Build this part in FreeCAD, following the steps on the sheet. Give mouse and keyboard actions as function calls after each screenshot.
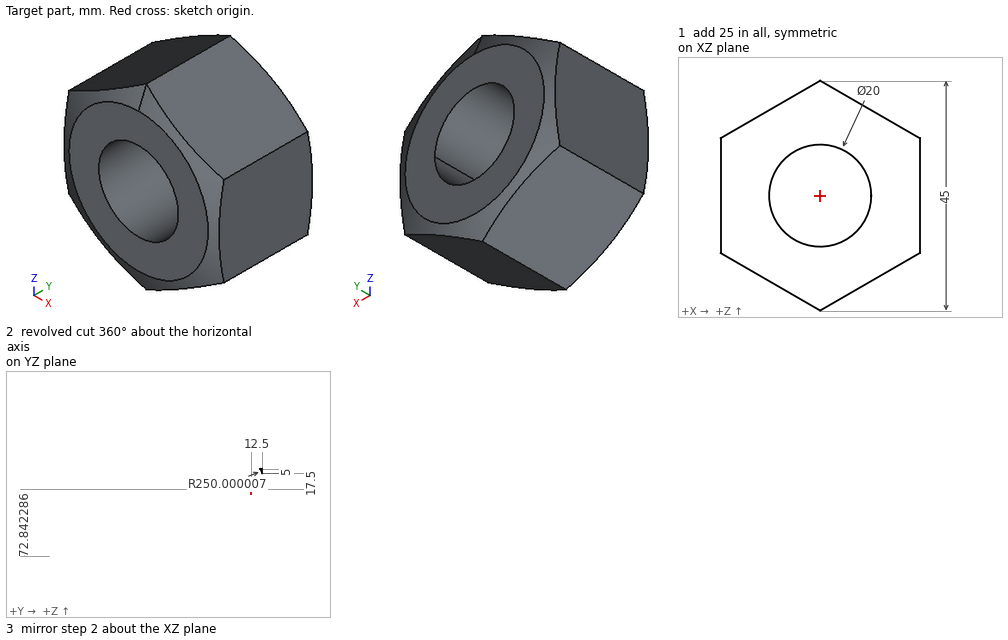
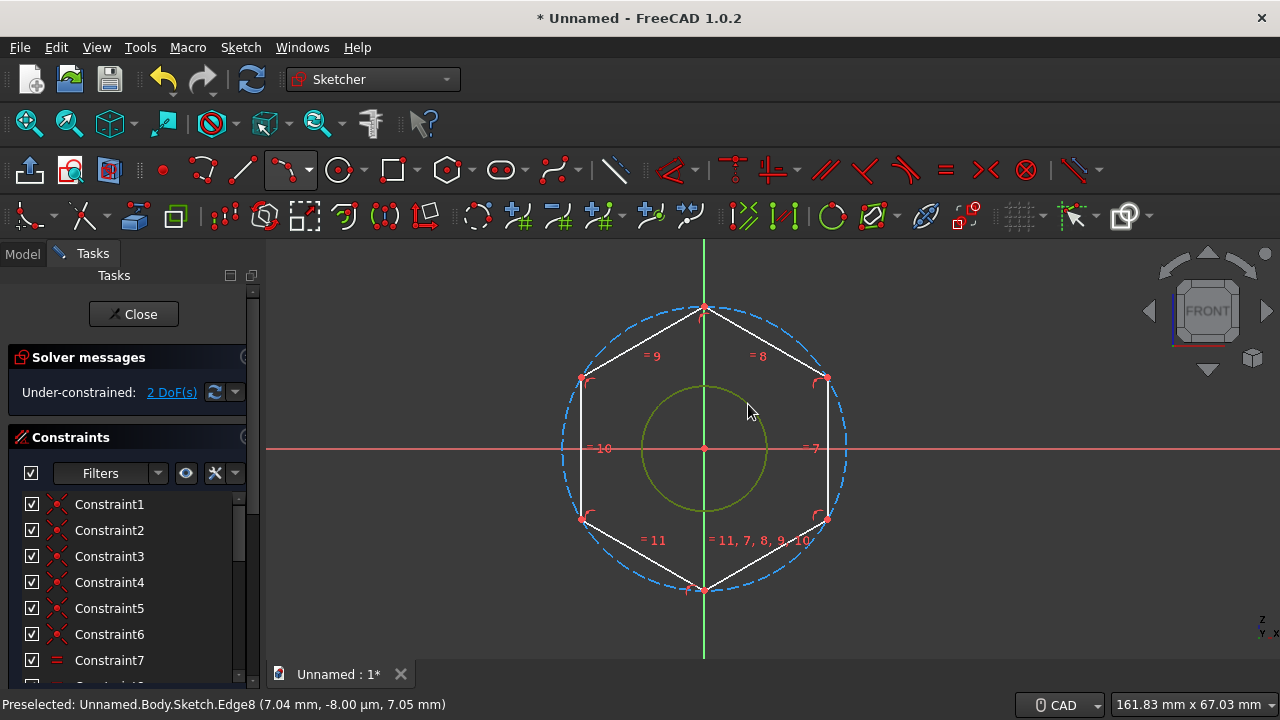
key(k)
key(o)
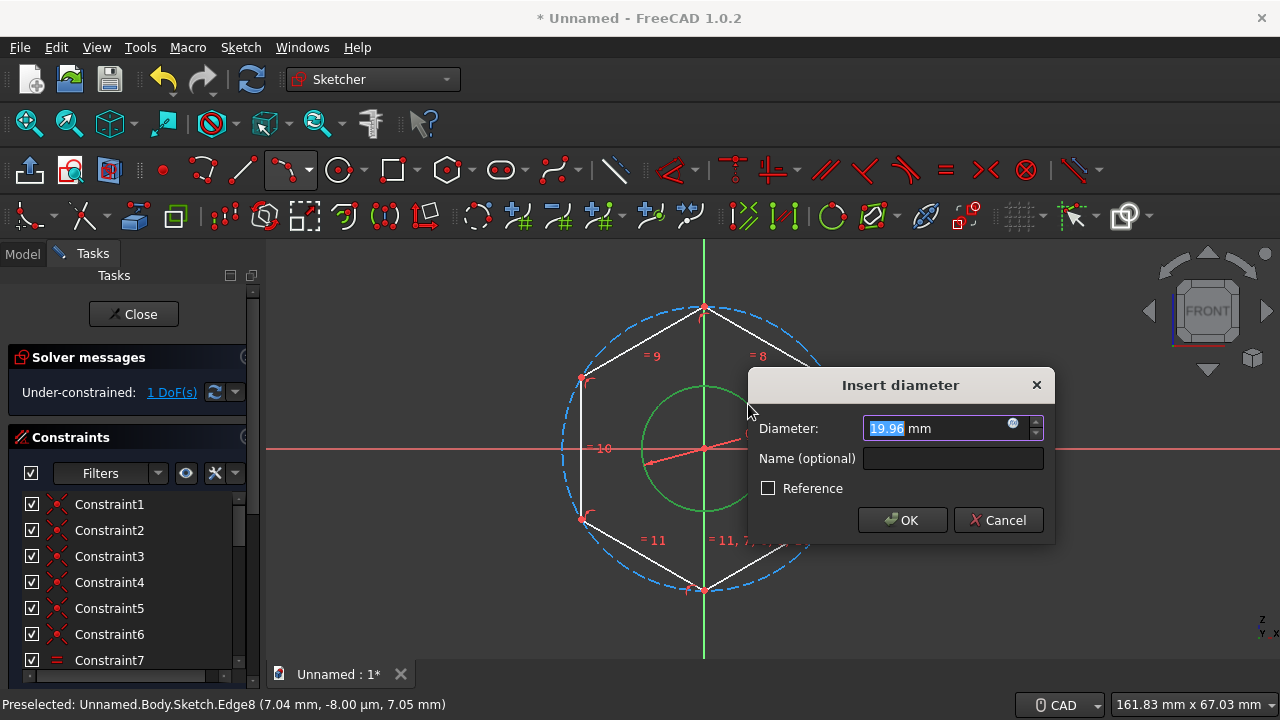
text(20)
key(Return)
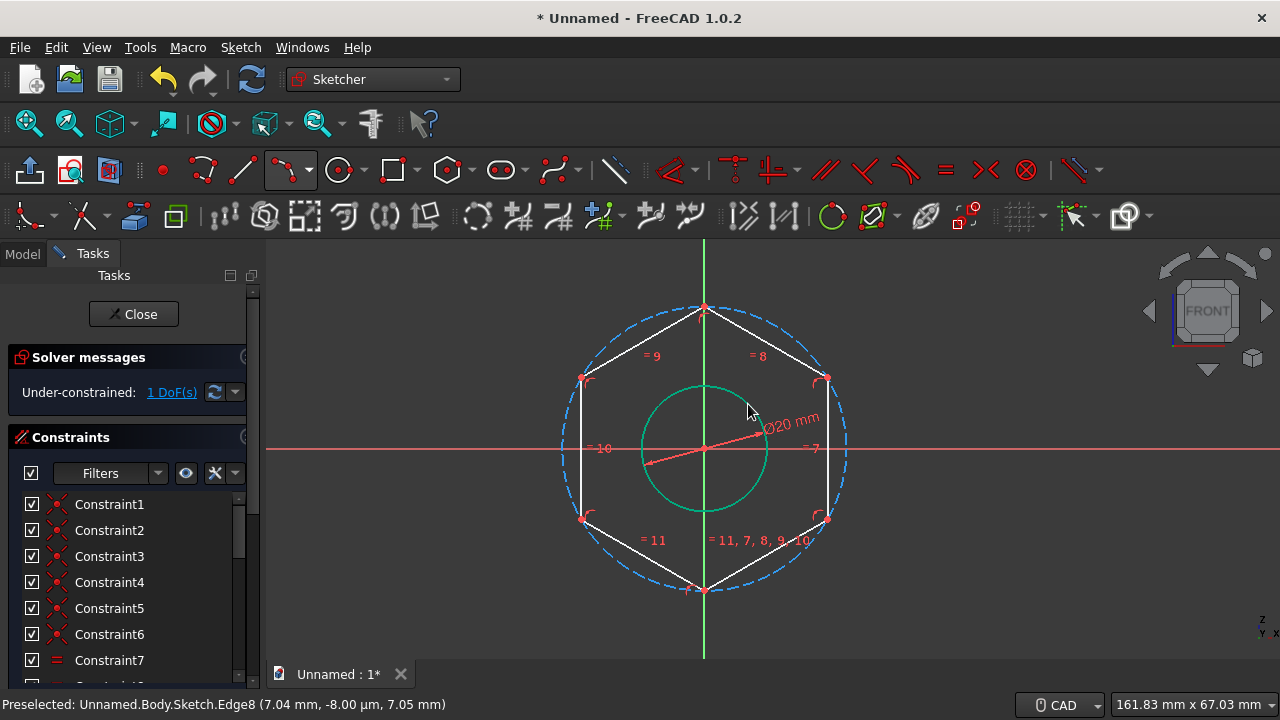
click(704, 591)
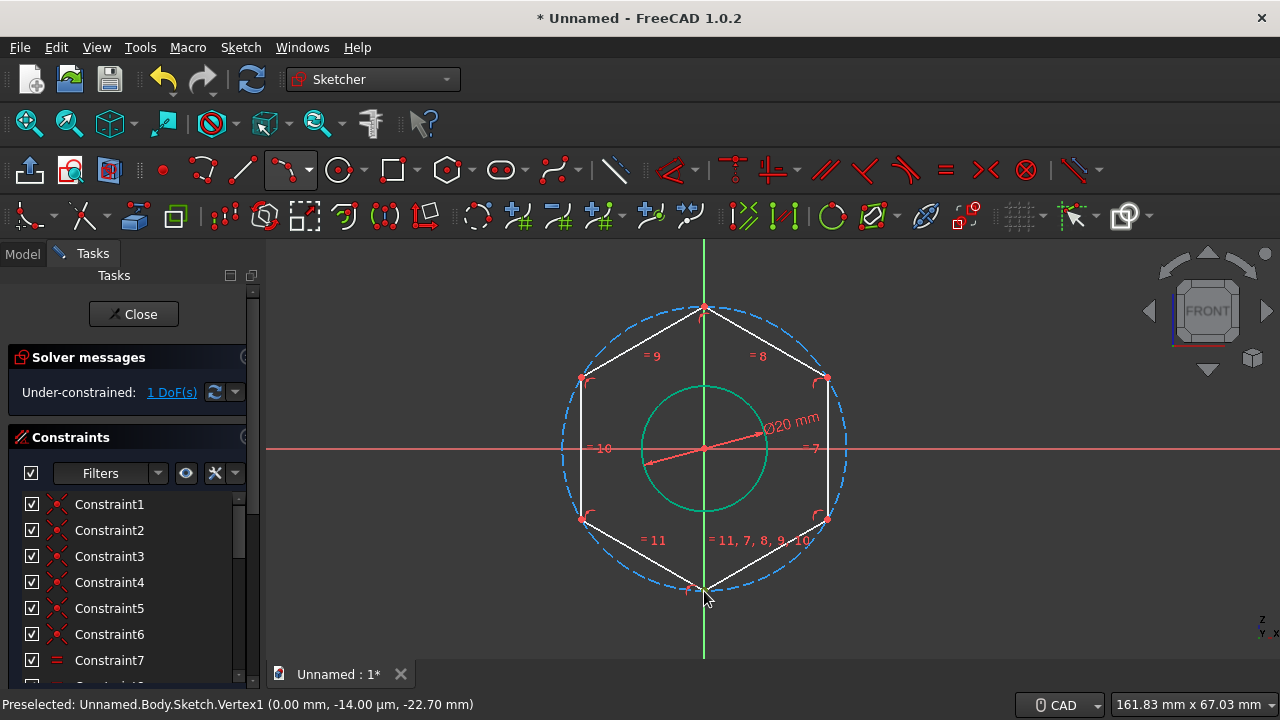
click(704, 307)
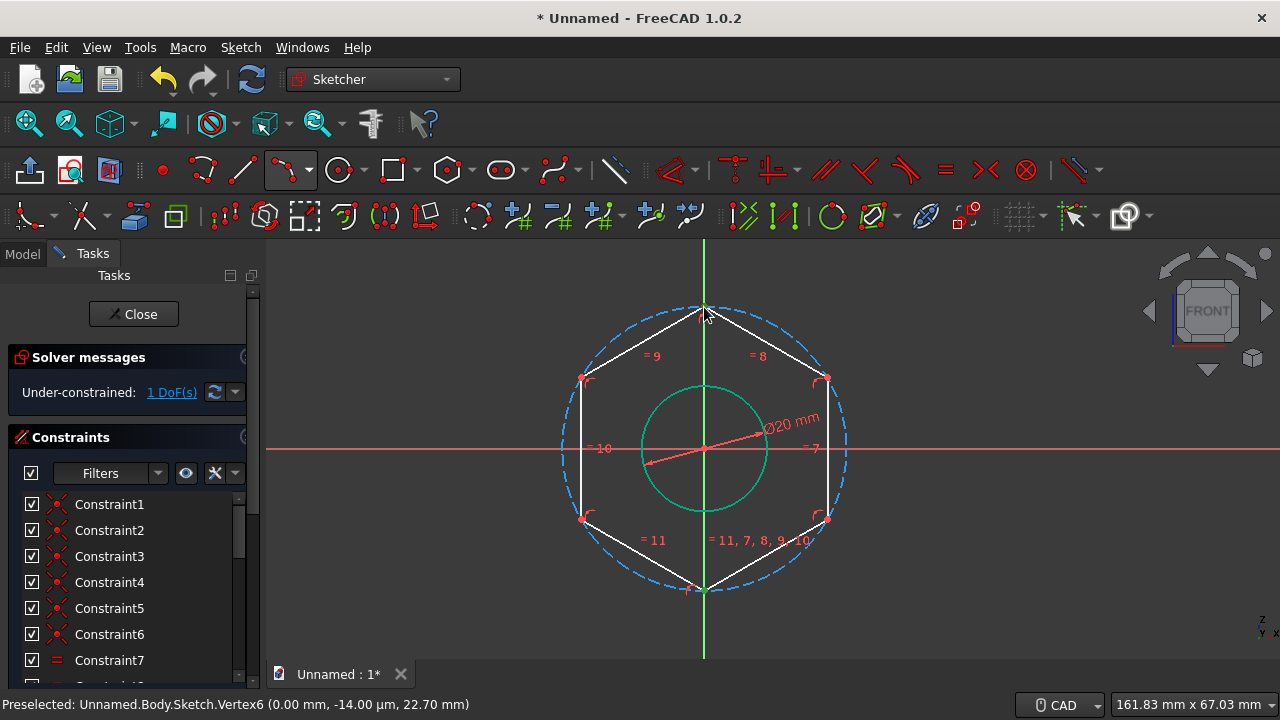
click(698, 170)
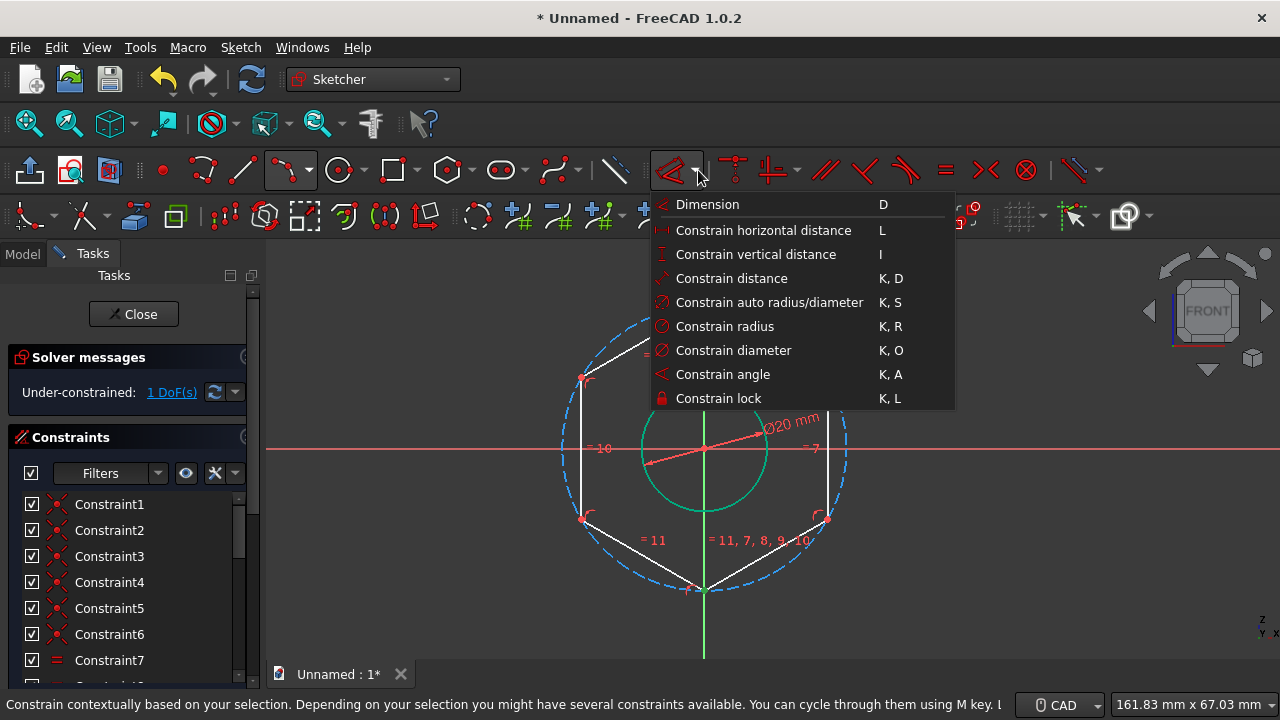
click(803, 254)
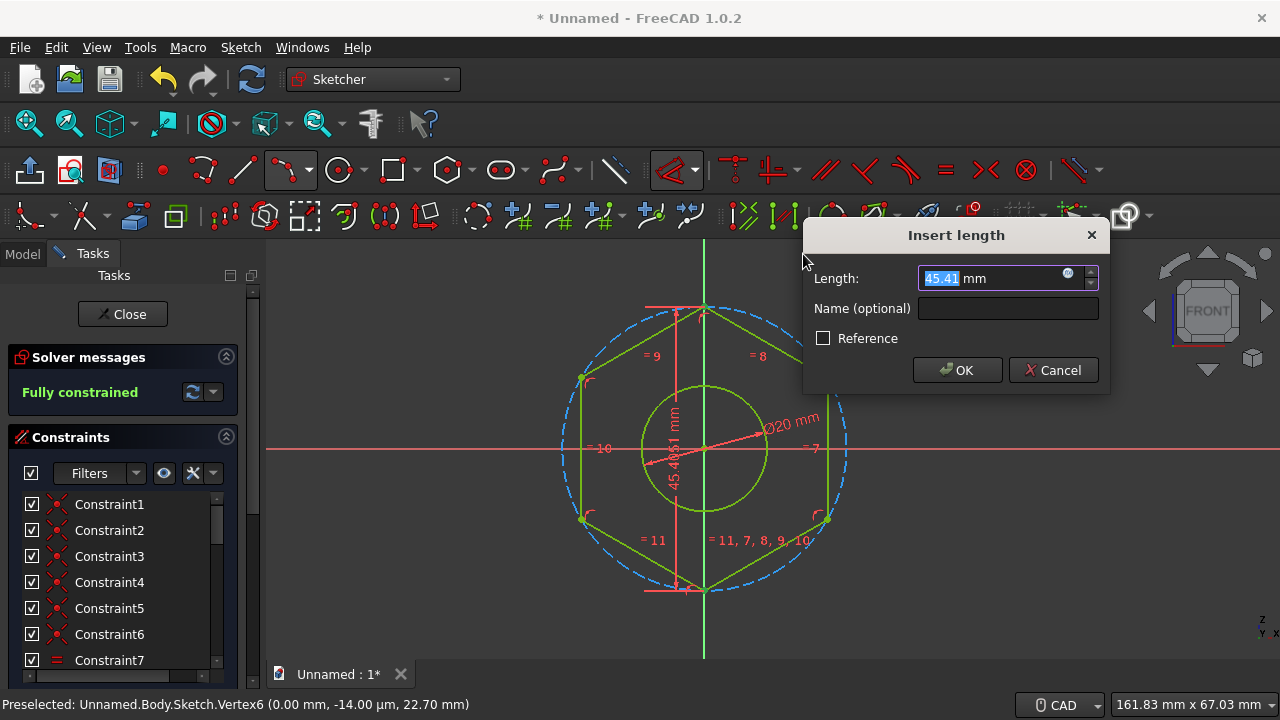
text(45)
key(Return)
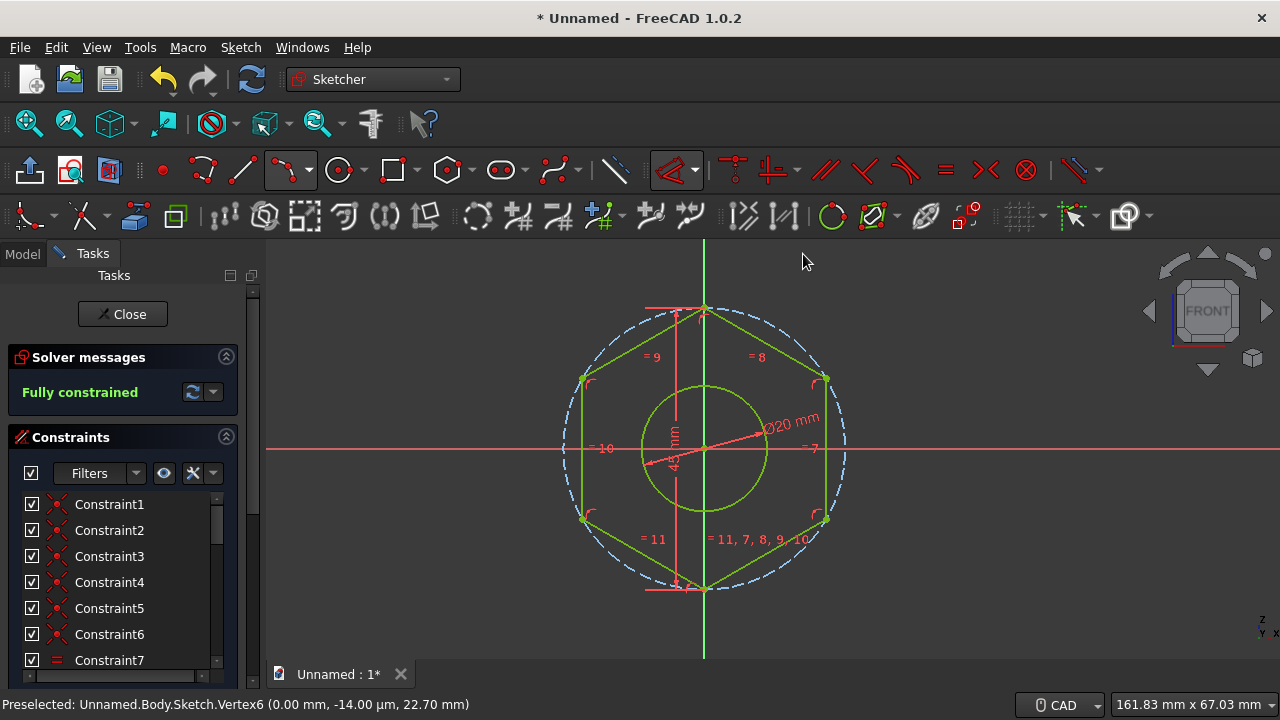
click(123, 314)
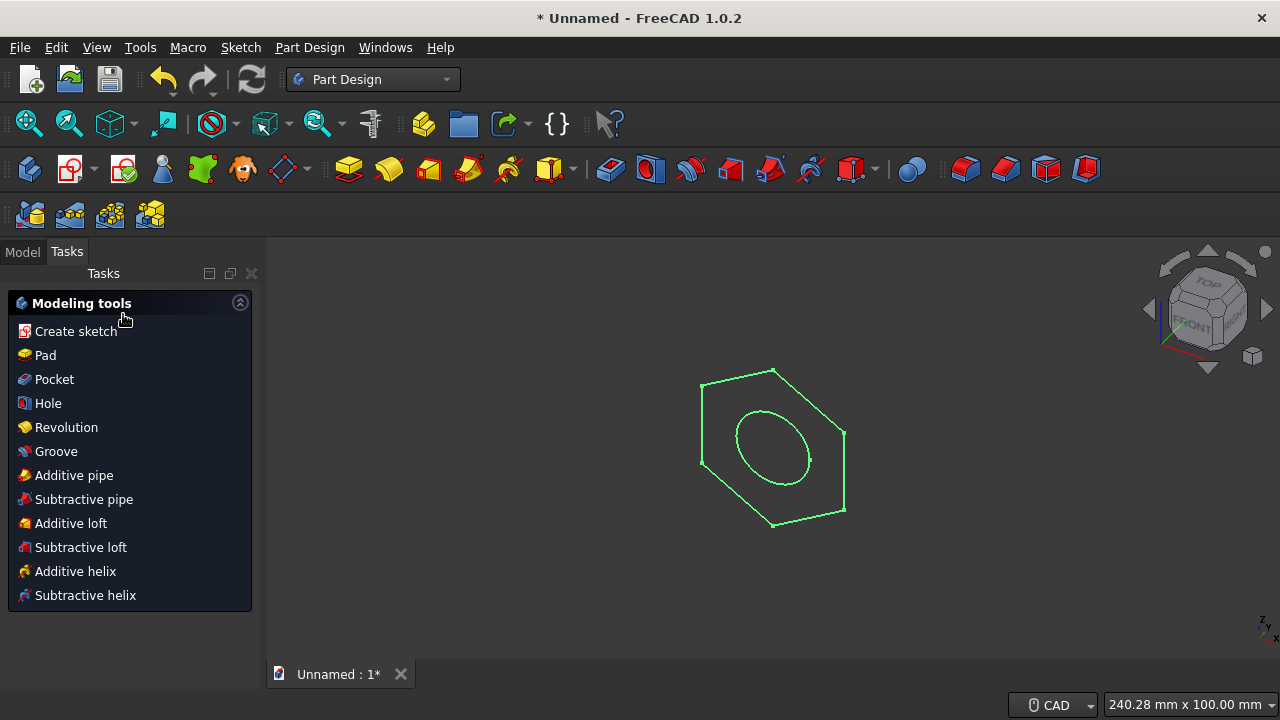
click(350, 170)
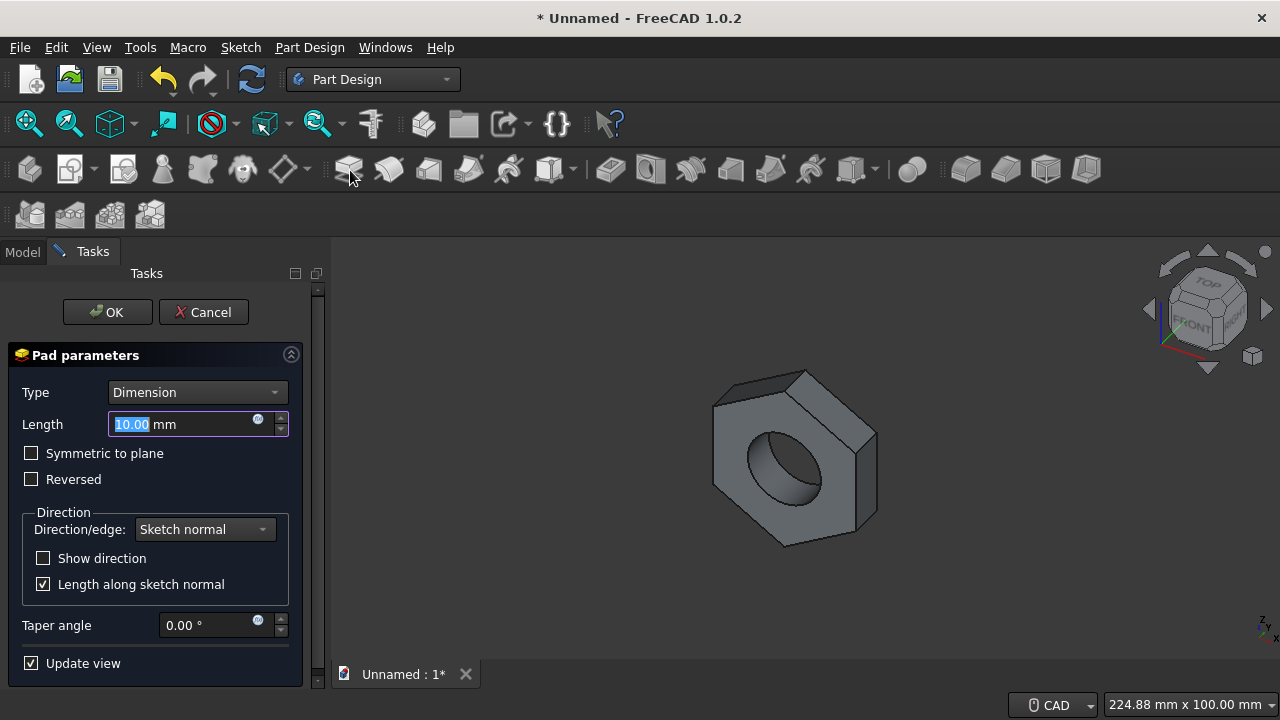
text(25)
key(Tab)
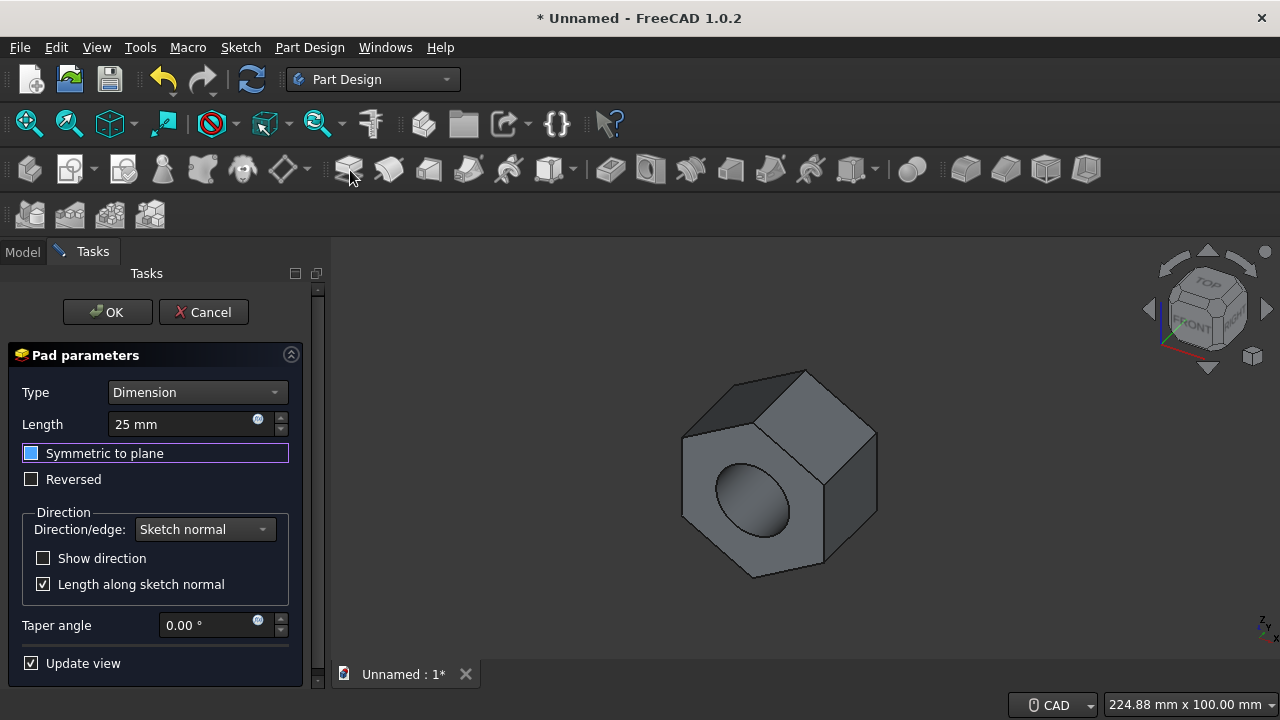
click(30, 453)